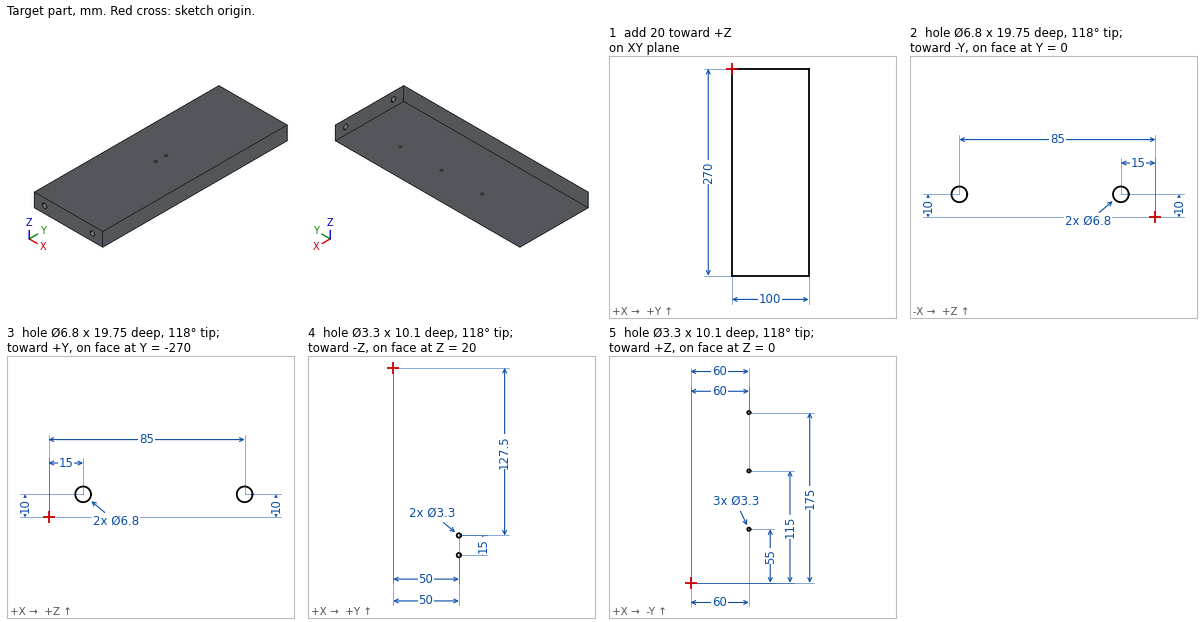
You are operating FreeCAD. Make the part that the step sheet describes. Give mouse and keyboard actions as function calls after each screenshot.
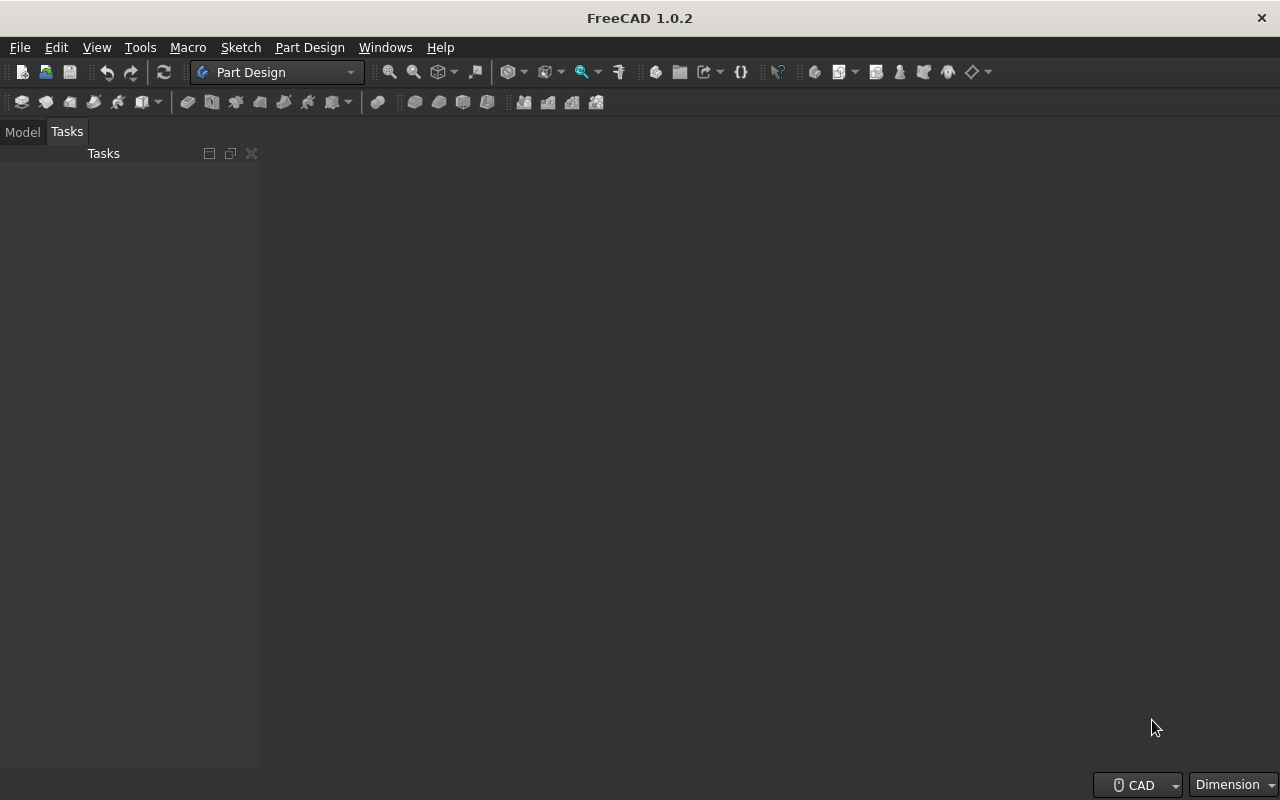
click(22, 72)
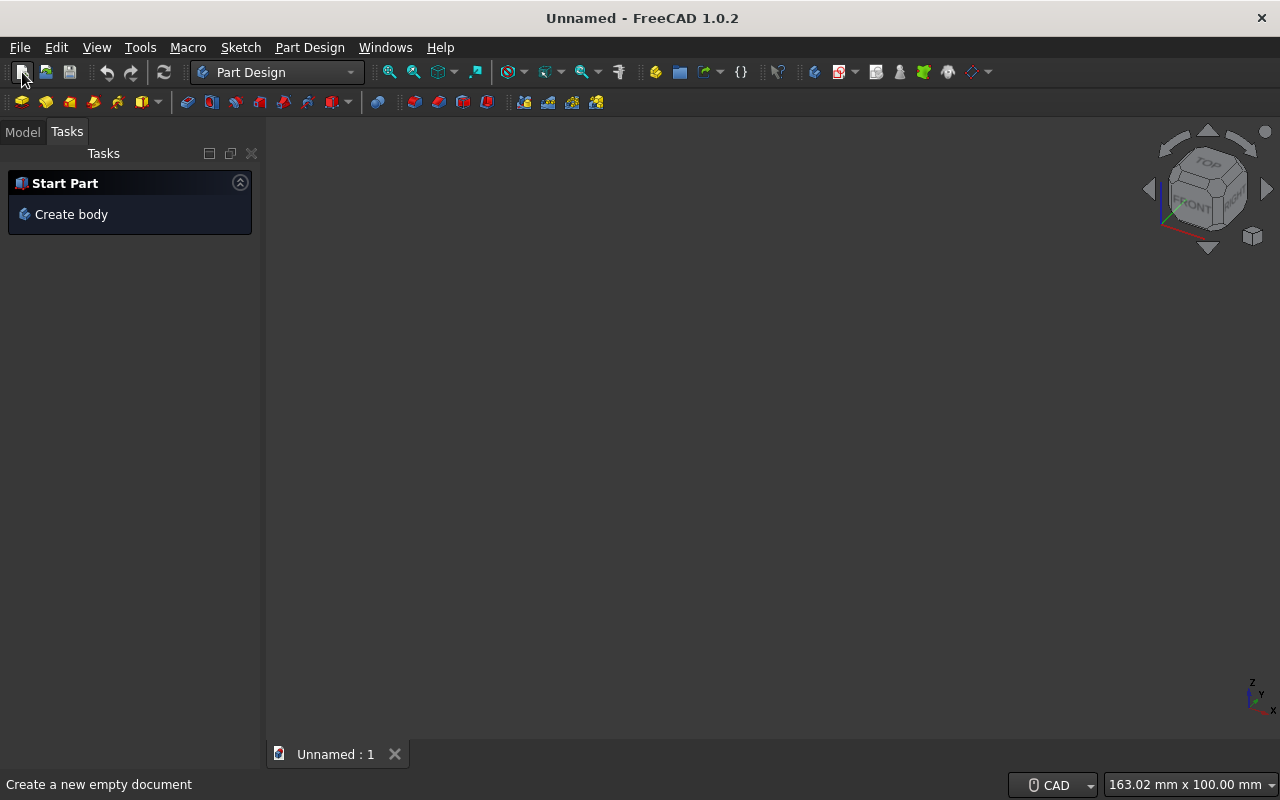
click(840, 72)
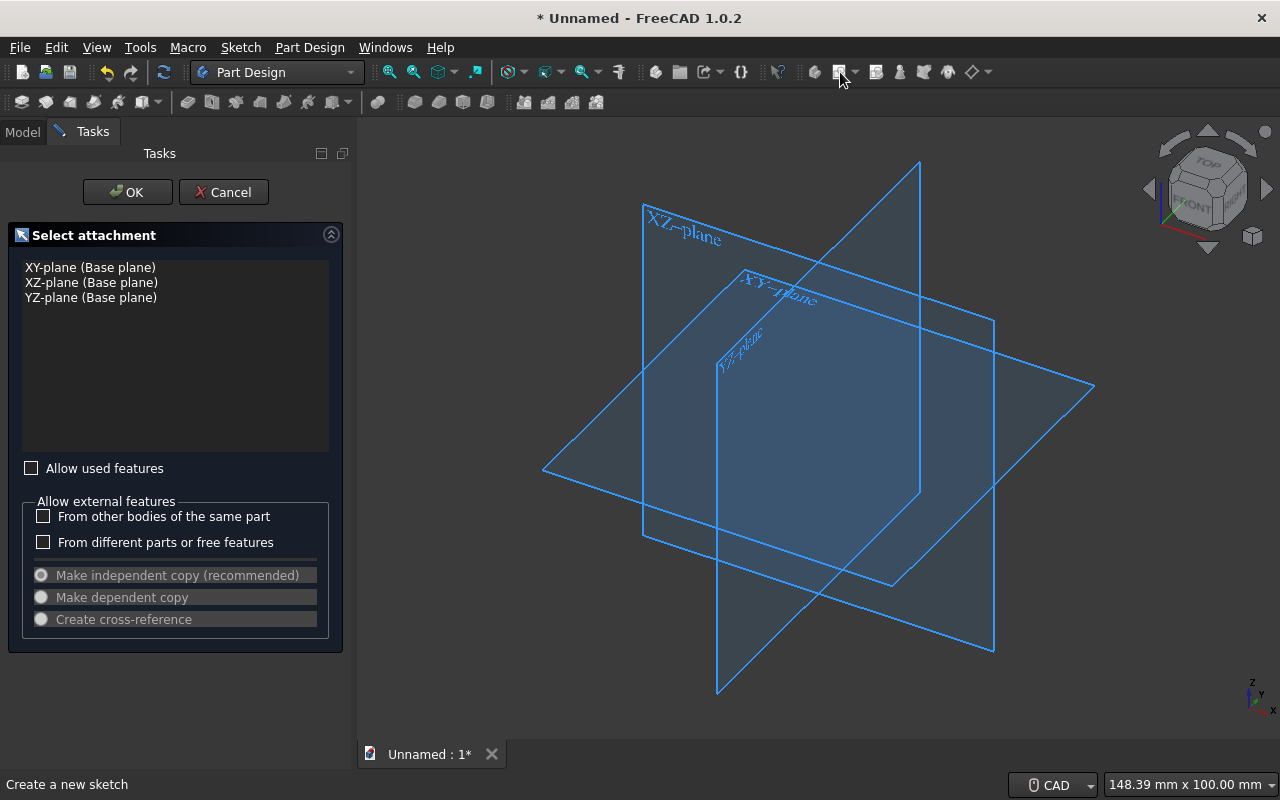
click(82, 268)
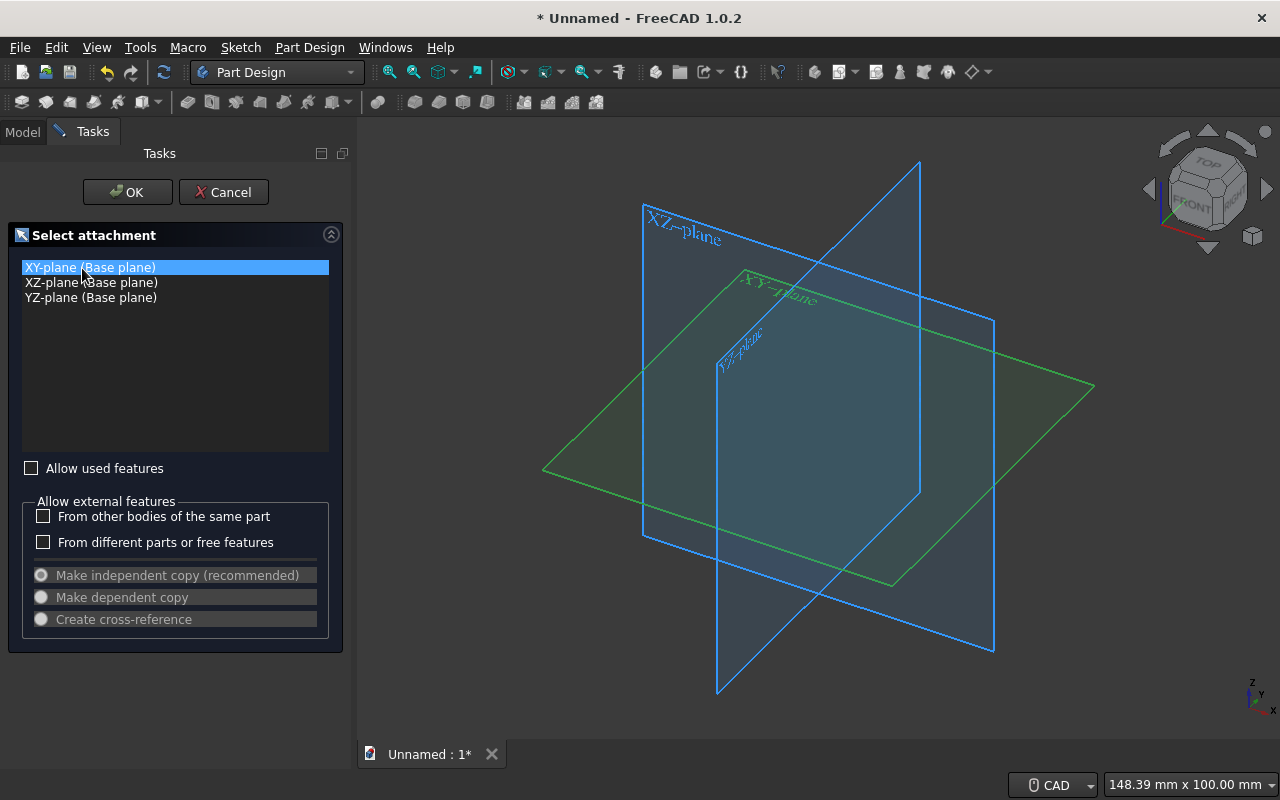
click(128, 192)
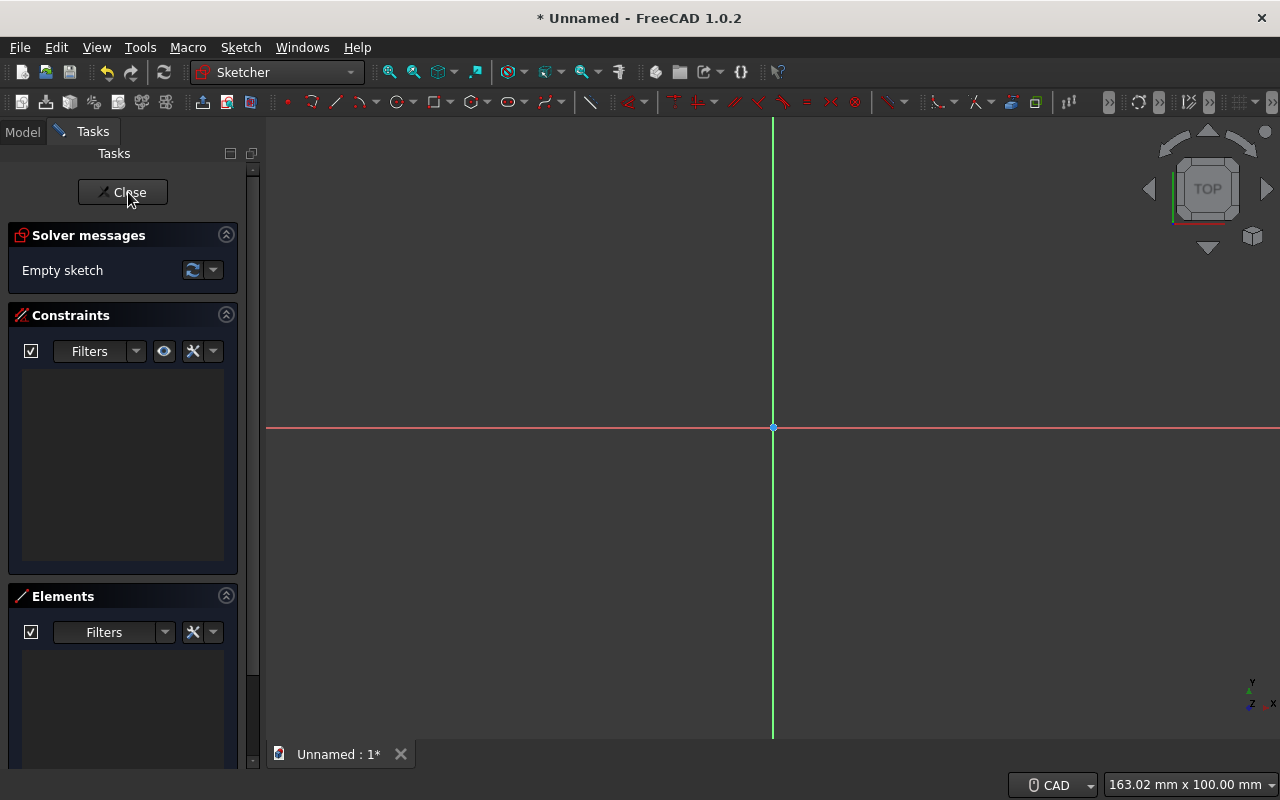
scroll(580, 153, down, 7)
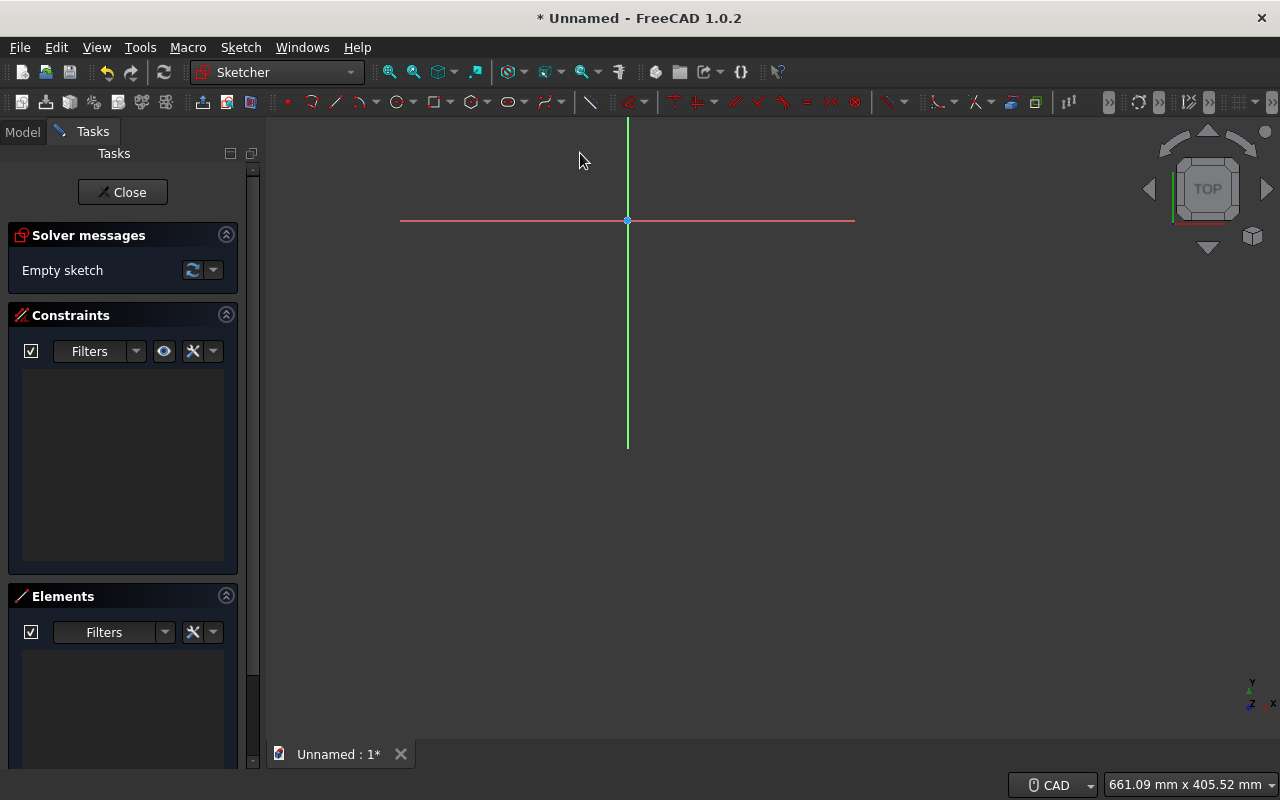
click(434, 102)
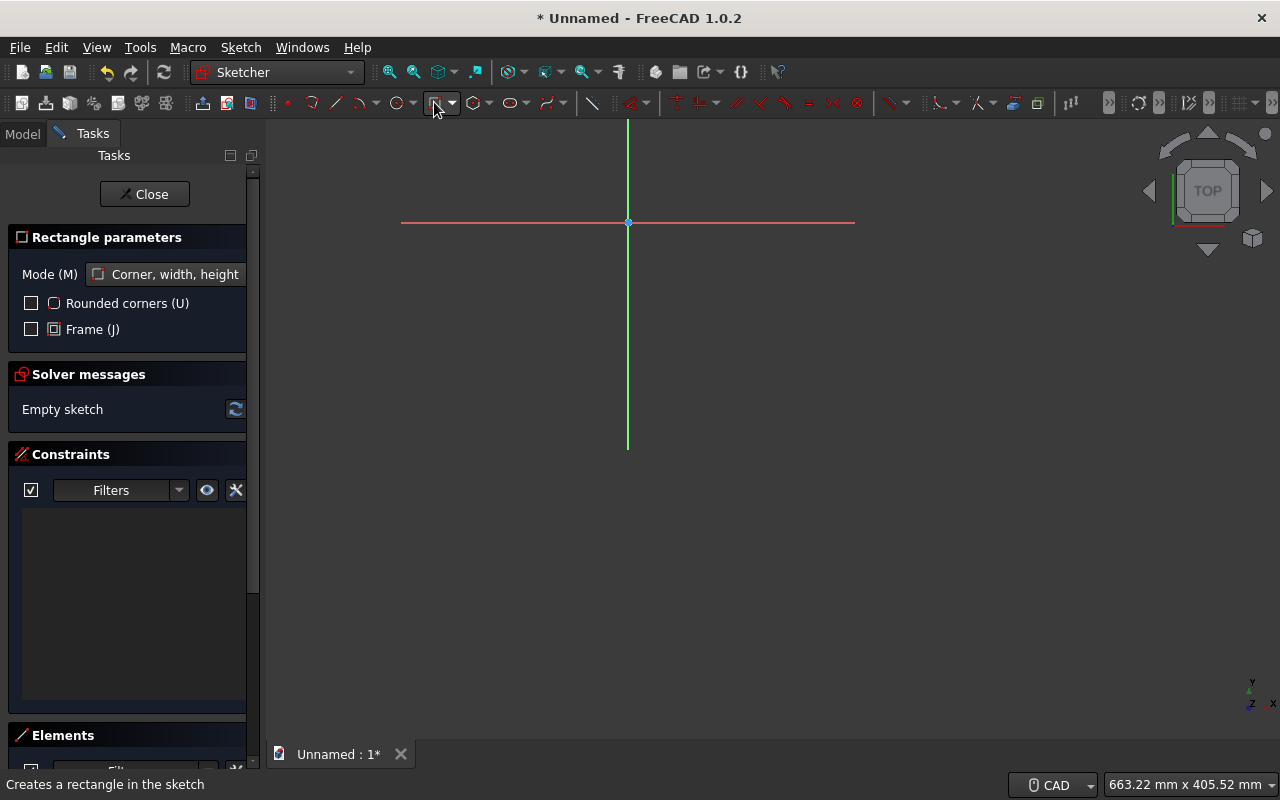
click(628, 223)
click(781, 635)
key(Escape)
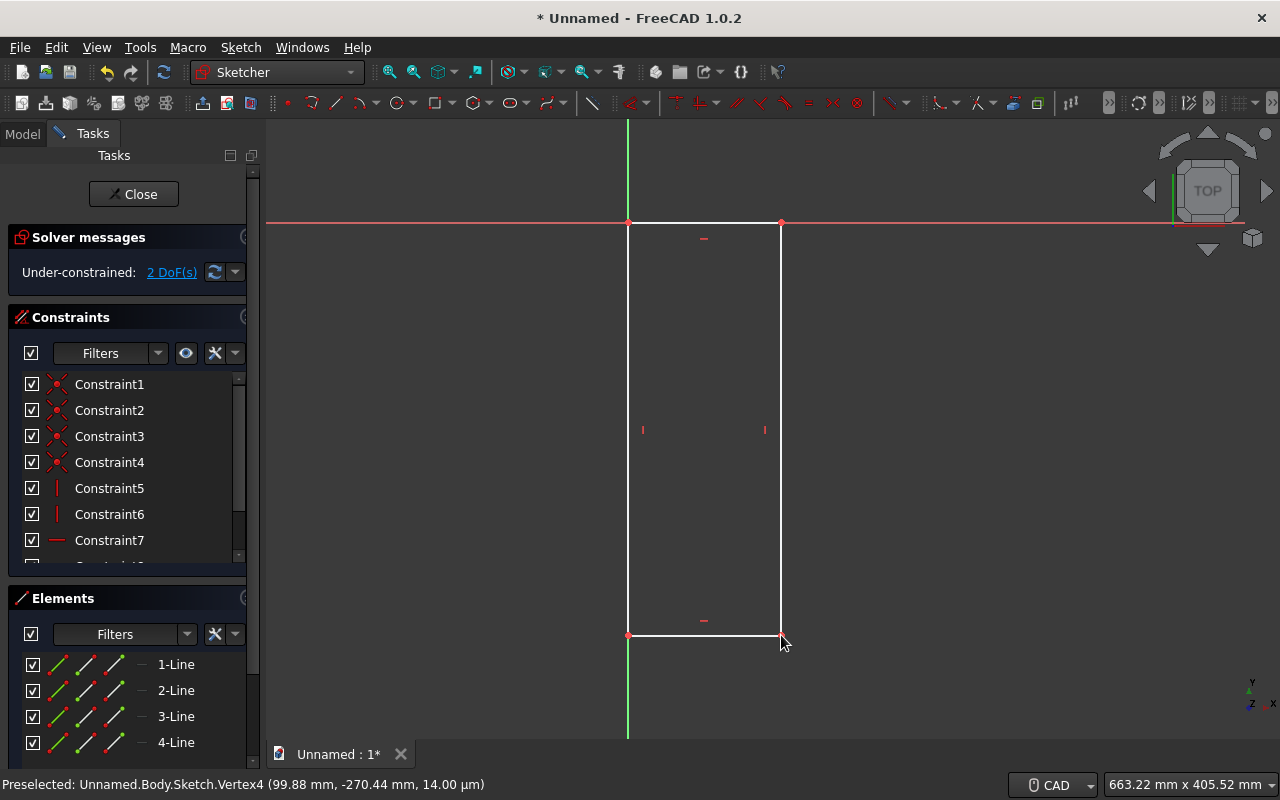
click(630, 104)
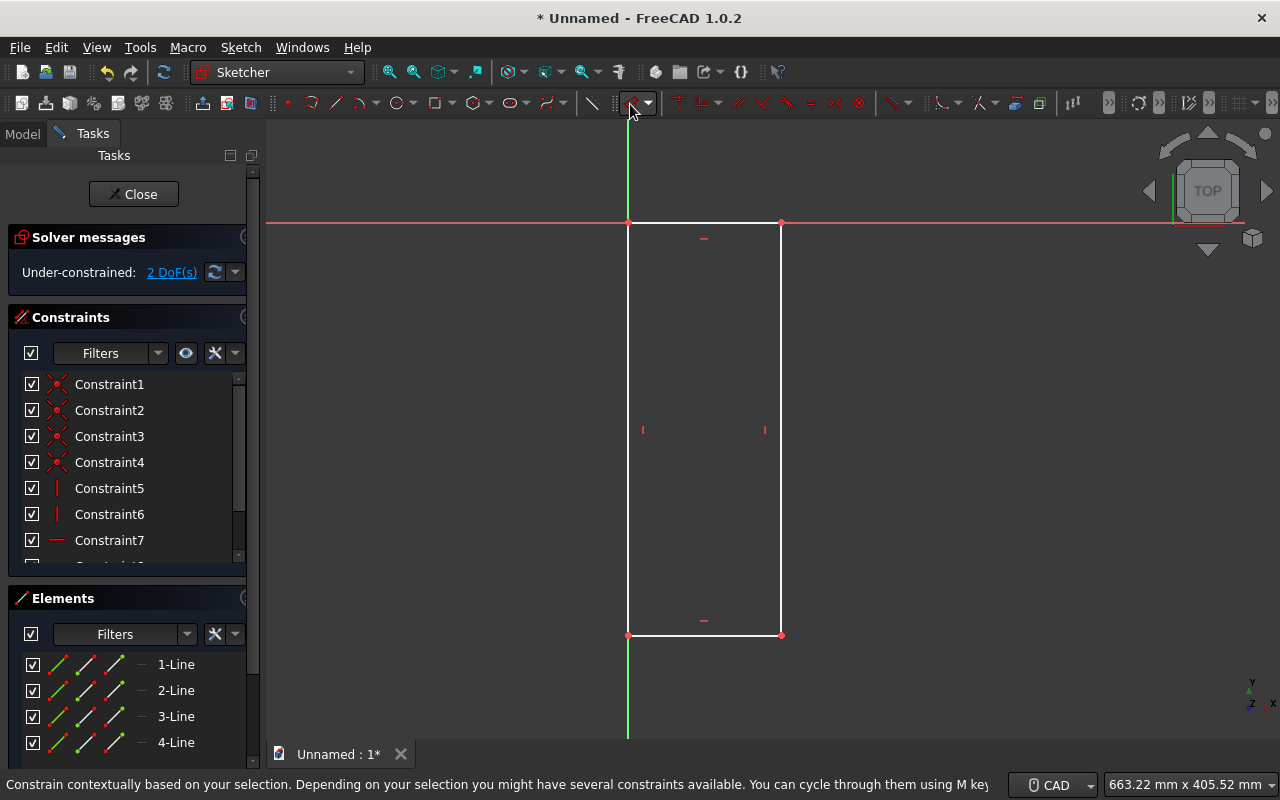
click(628, 347)
click(594, 429)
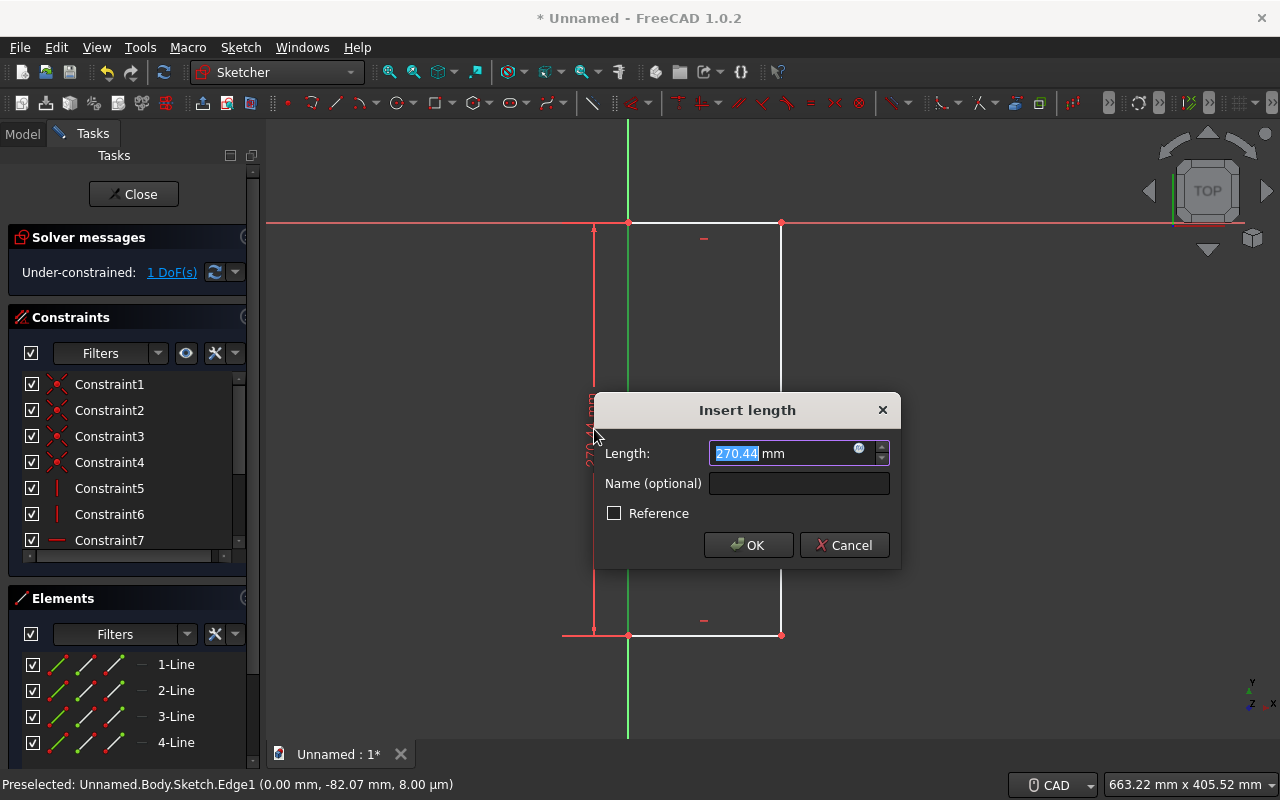
text(270)
key(Return)